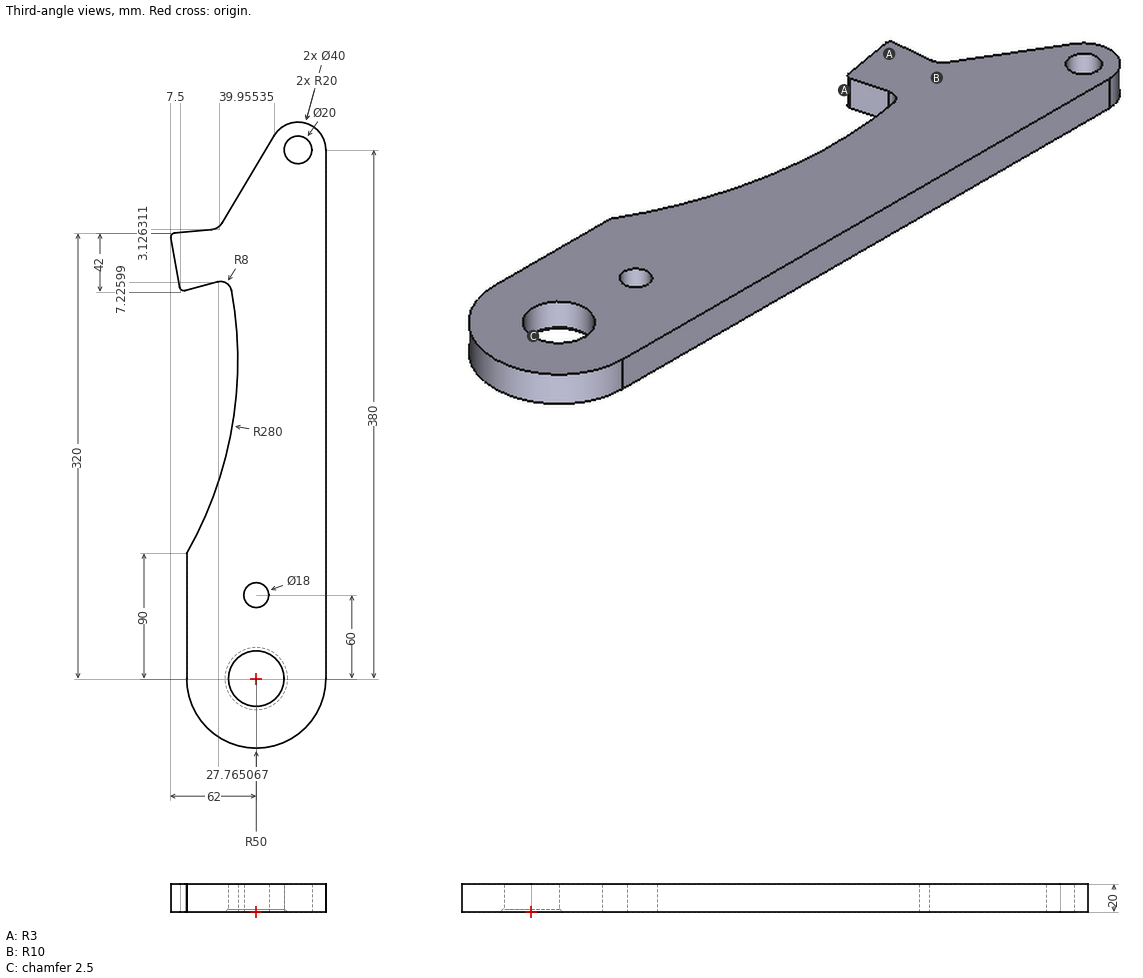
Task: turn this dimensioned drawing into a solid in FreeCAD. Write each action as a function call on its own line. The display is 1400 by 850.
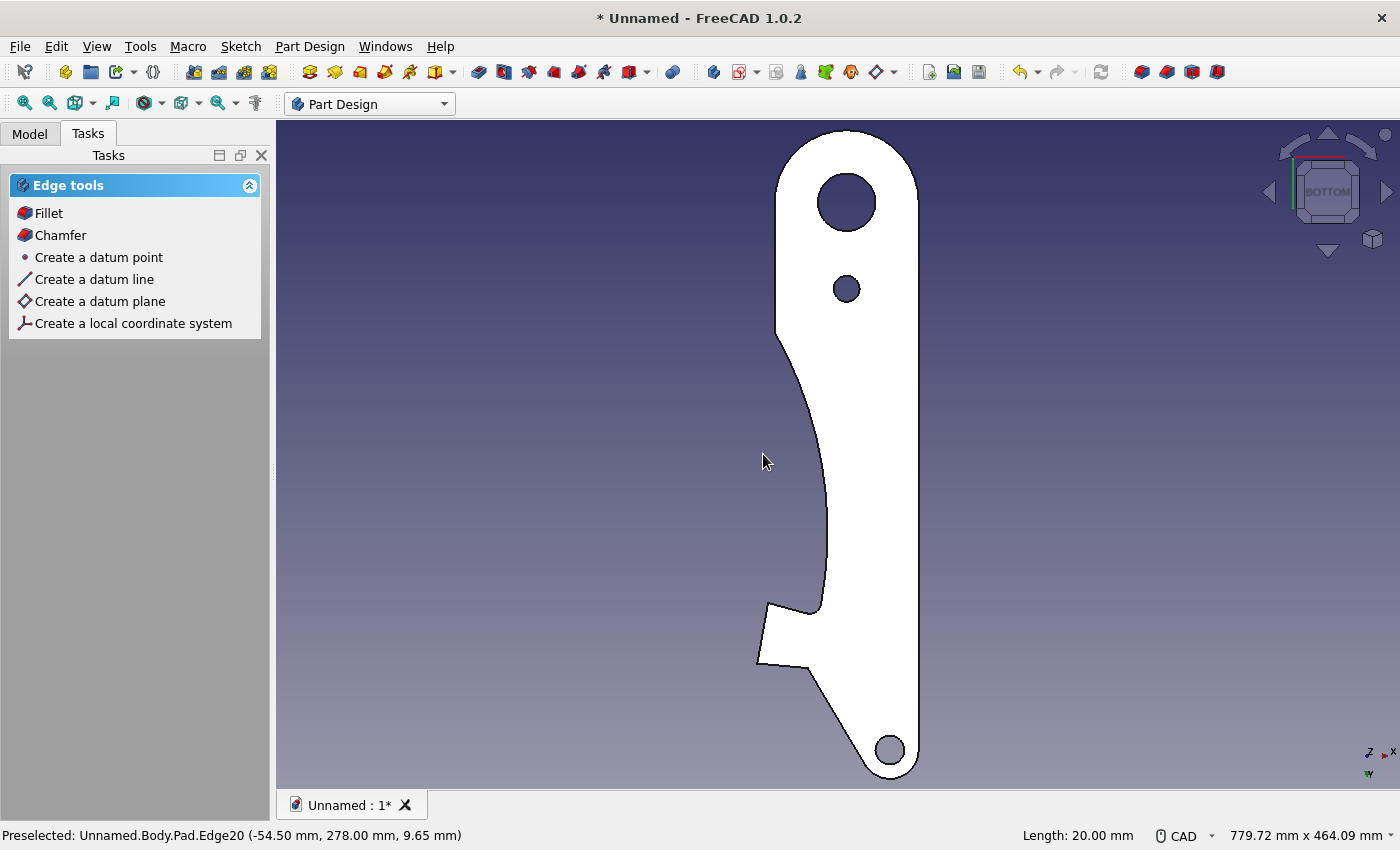
key(4)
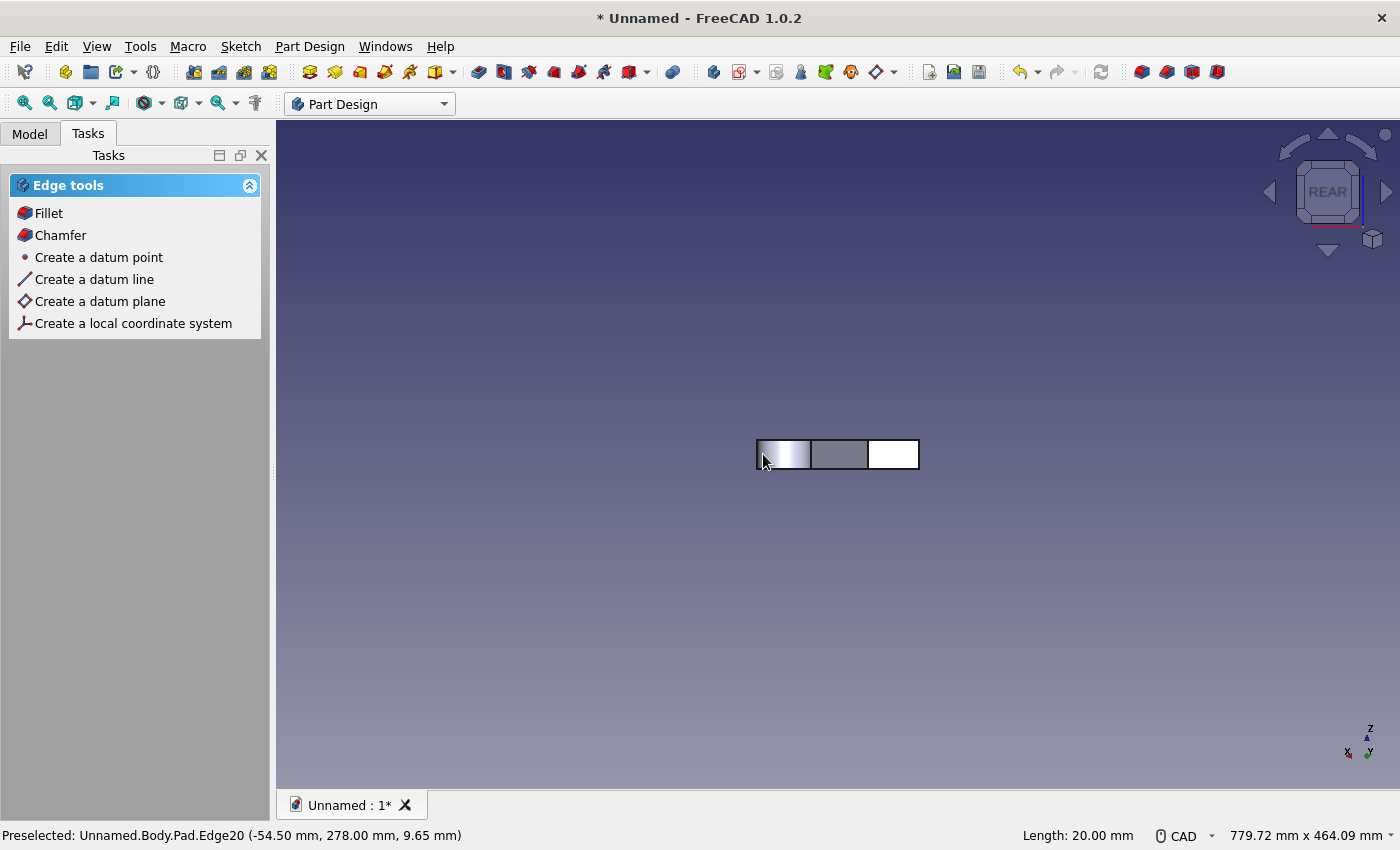
click(25, 104)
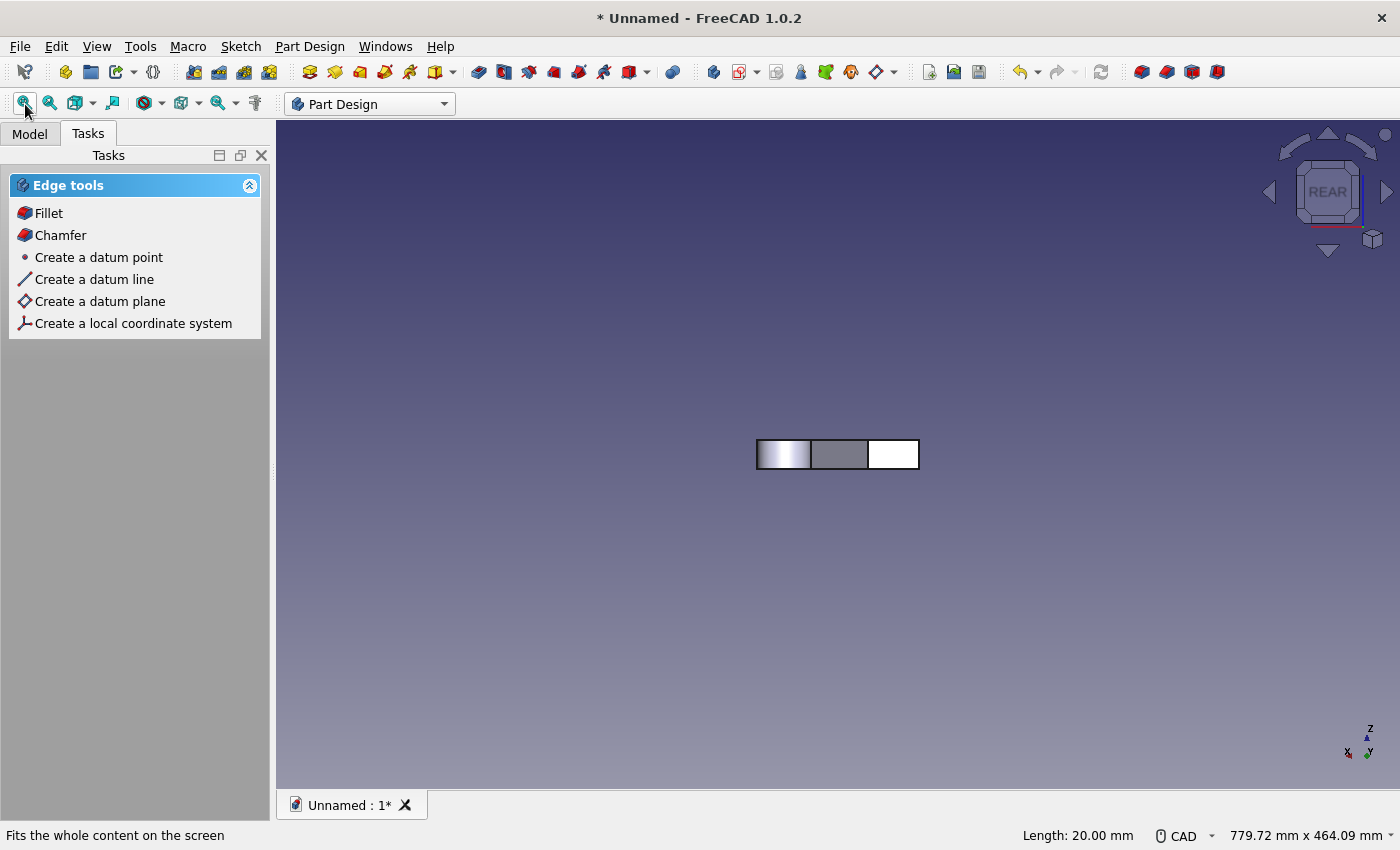
key(6)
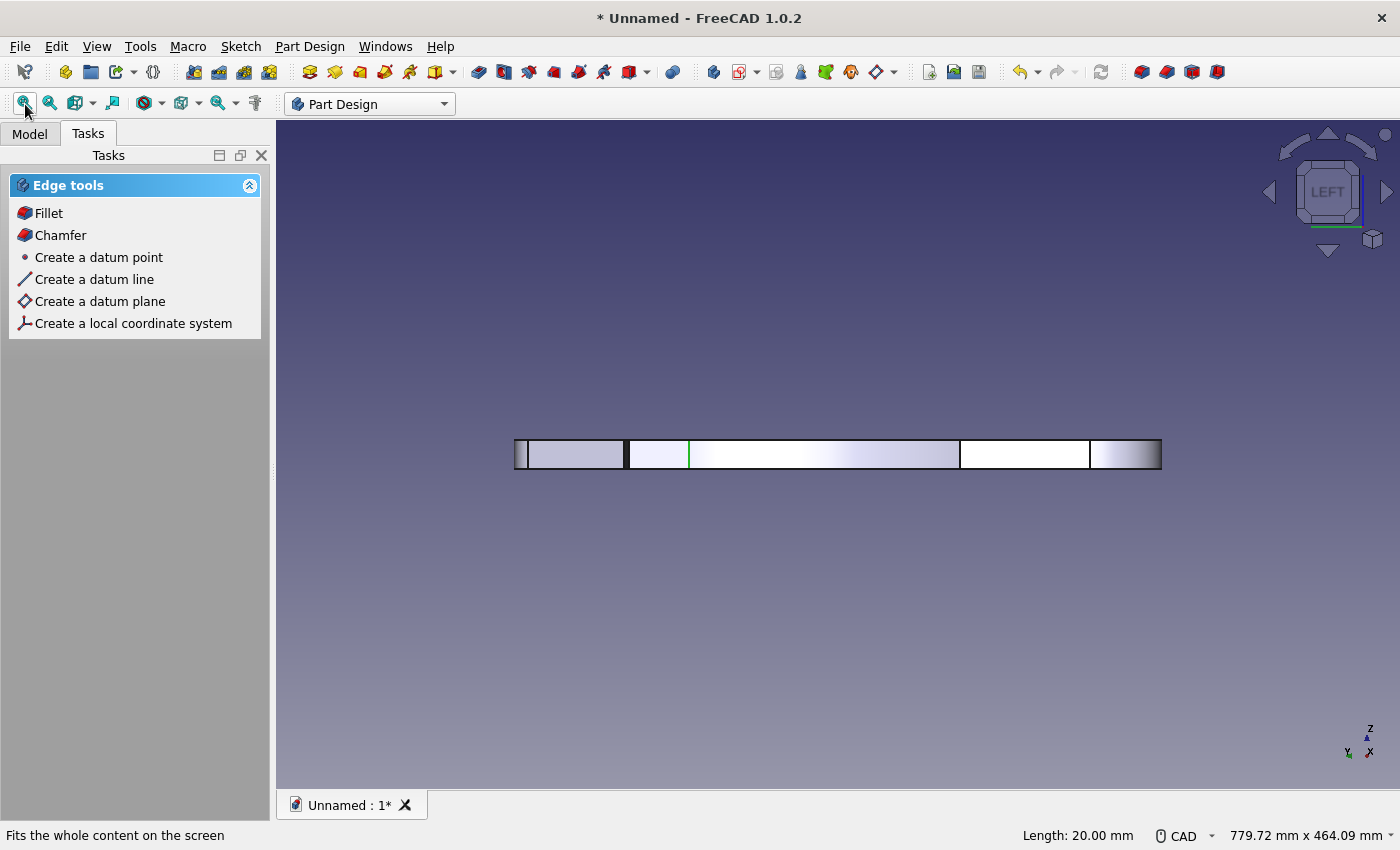
click(629, 453, ctrl)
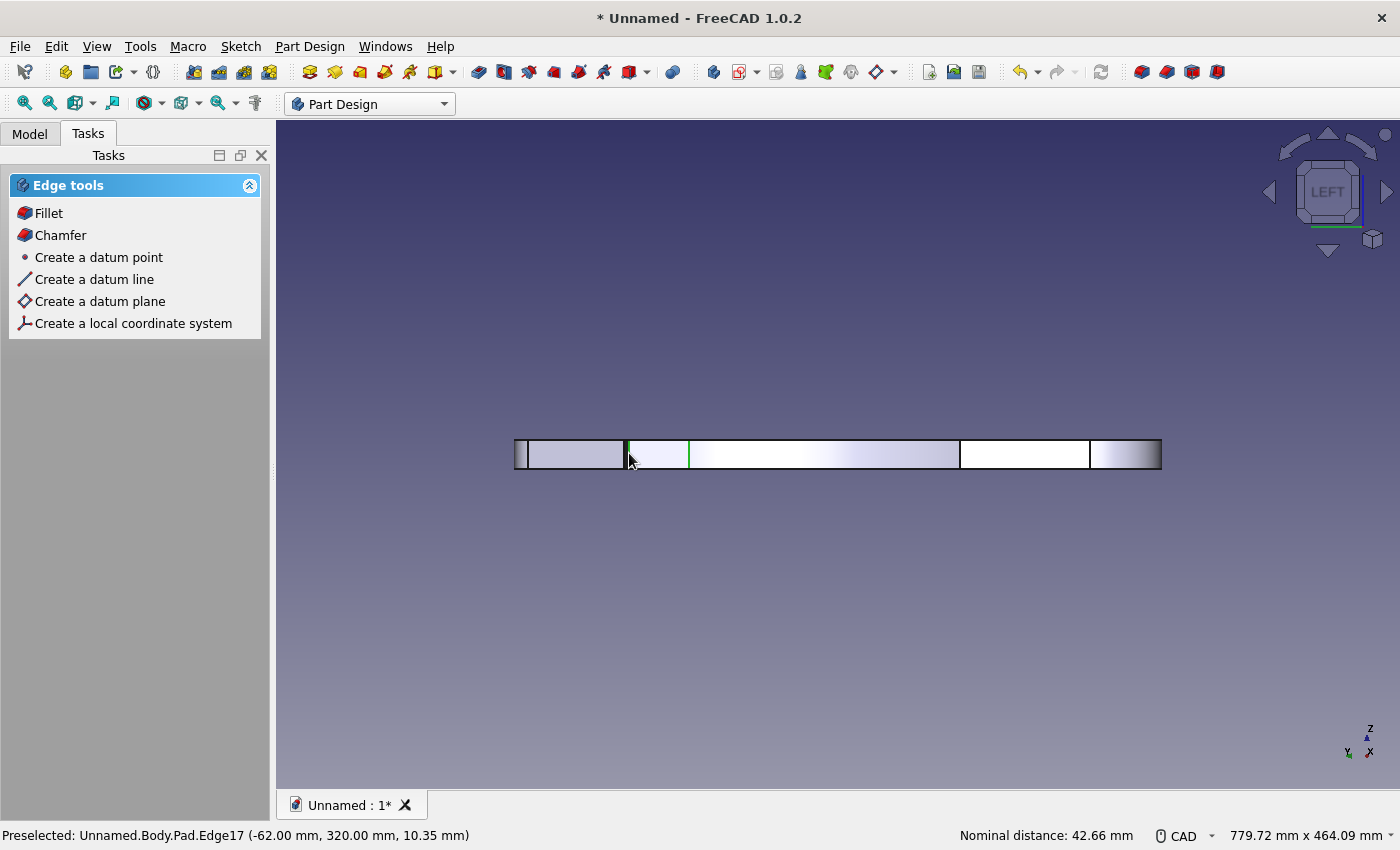
click(1142, 72)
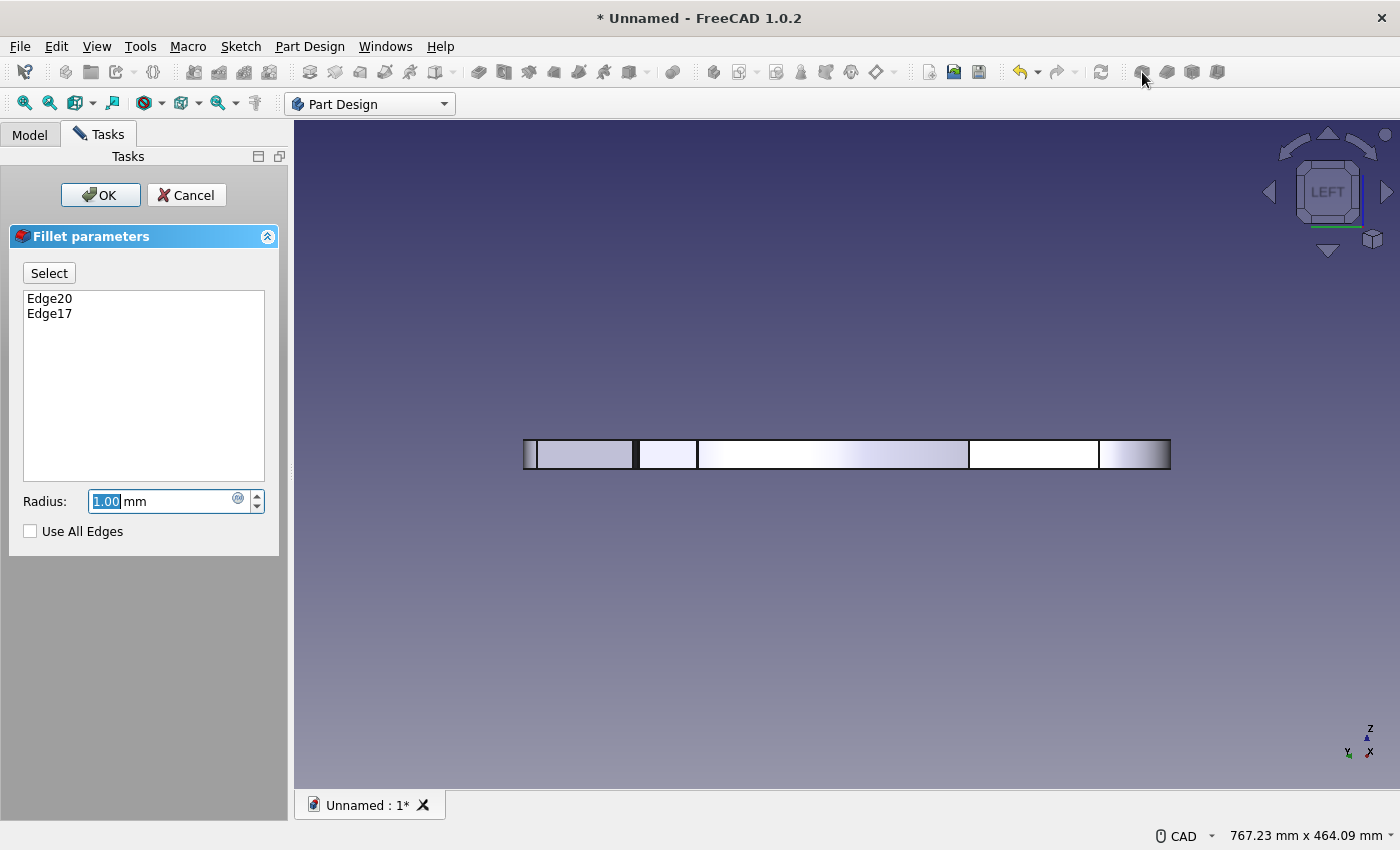
text(3)
key(Tab)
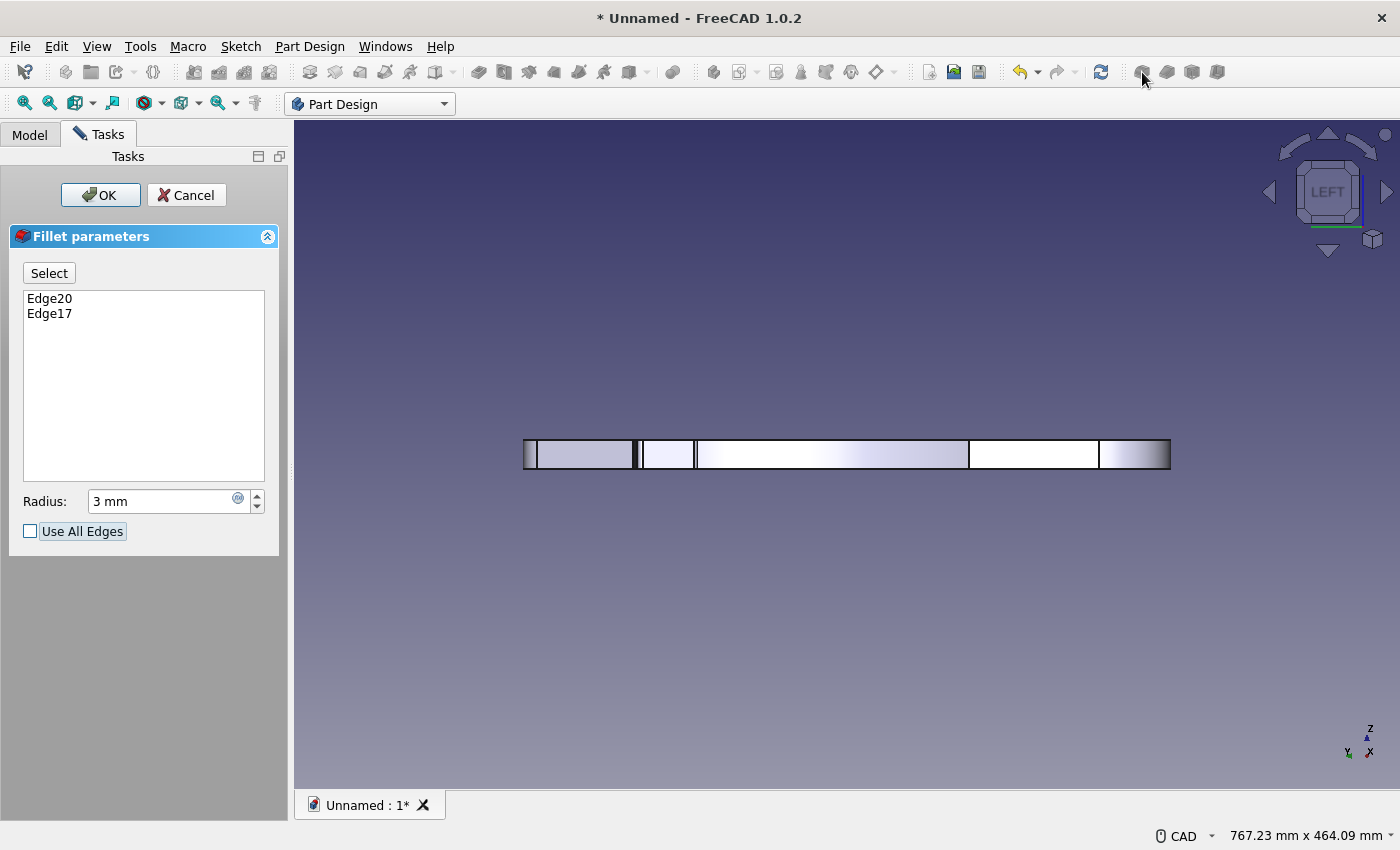
click(101, 195)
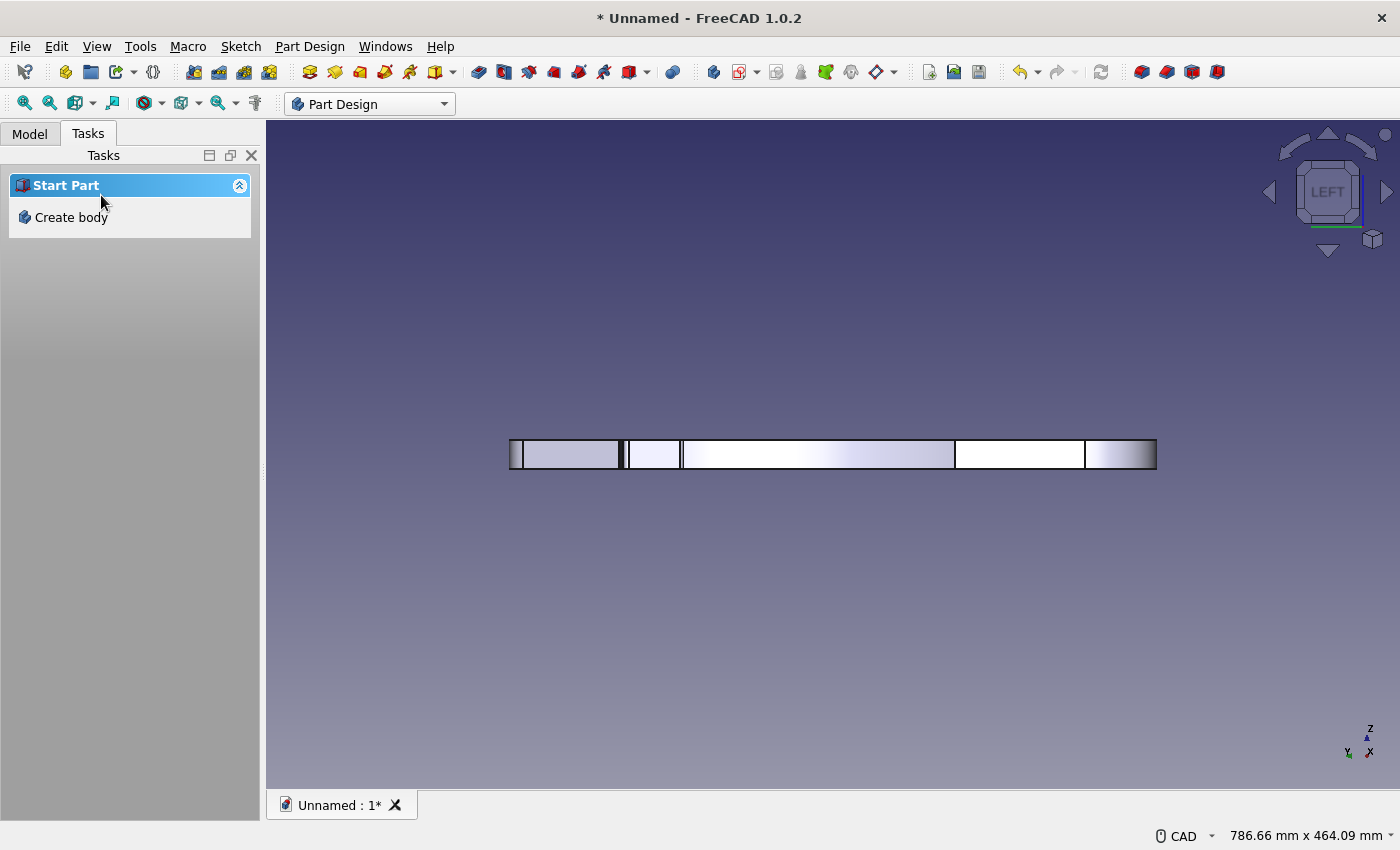
key(0)